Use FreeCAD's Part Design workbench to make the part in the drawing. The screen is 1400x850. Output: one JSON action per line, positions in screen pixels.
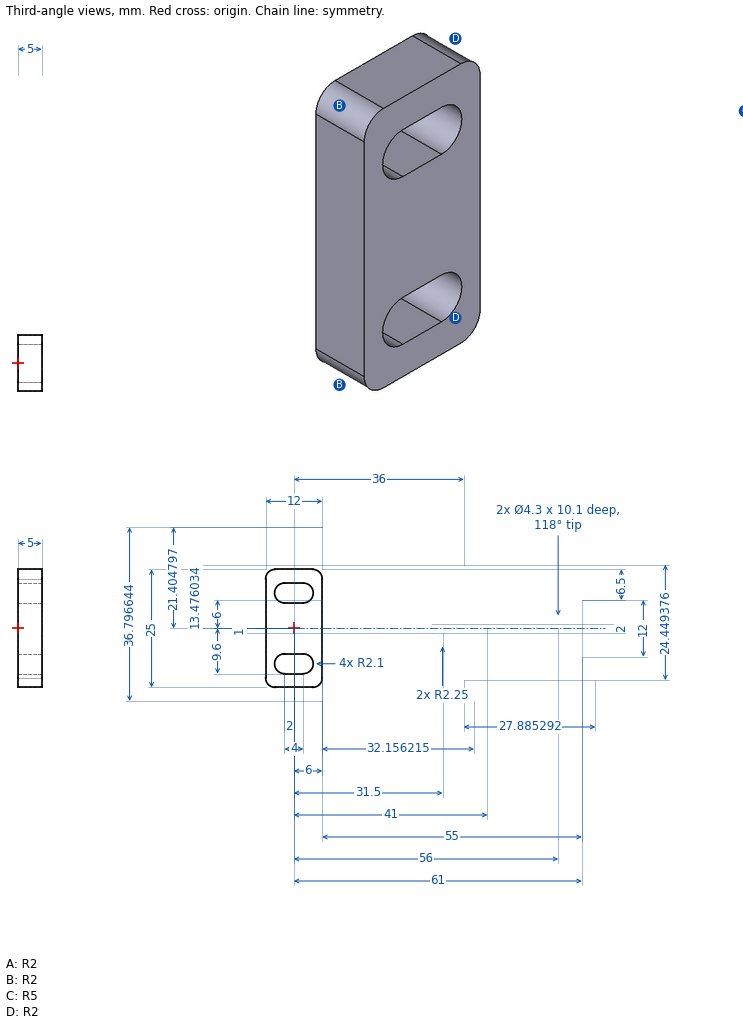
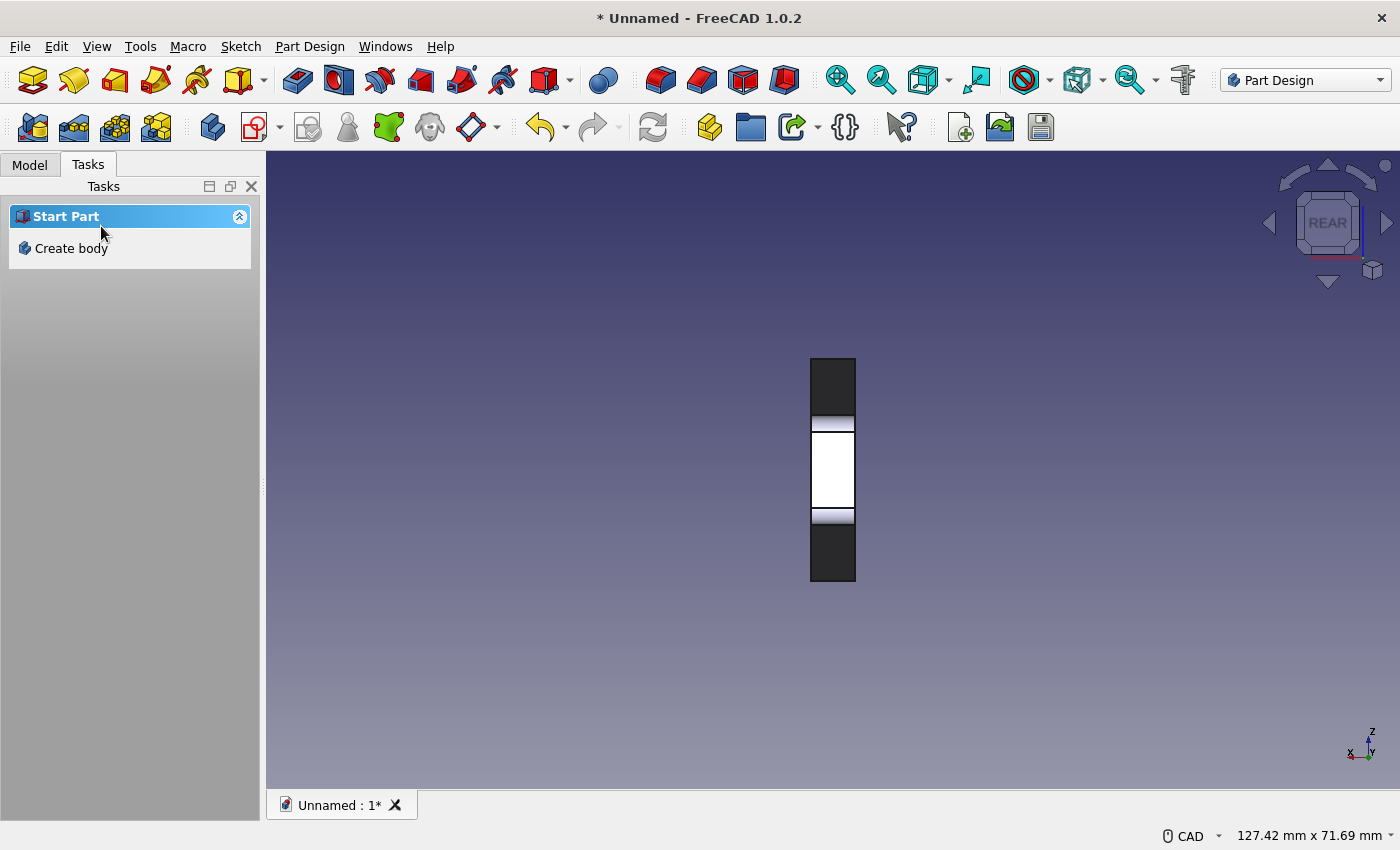
{"action": "left_click", "coordinate": [841, 80]}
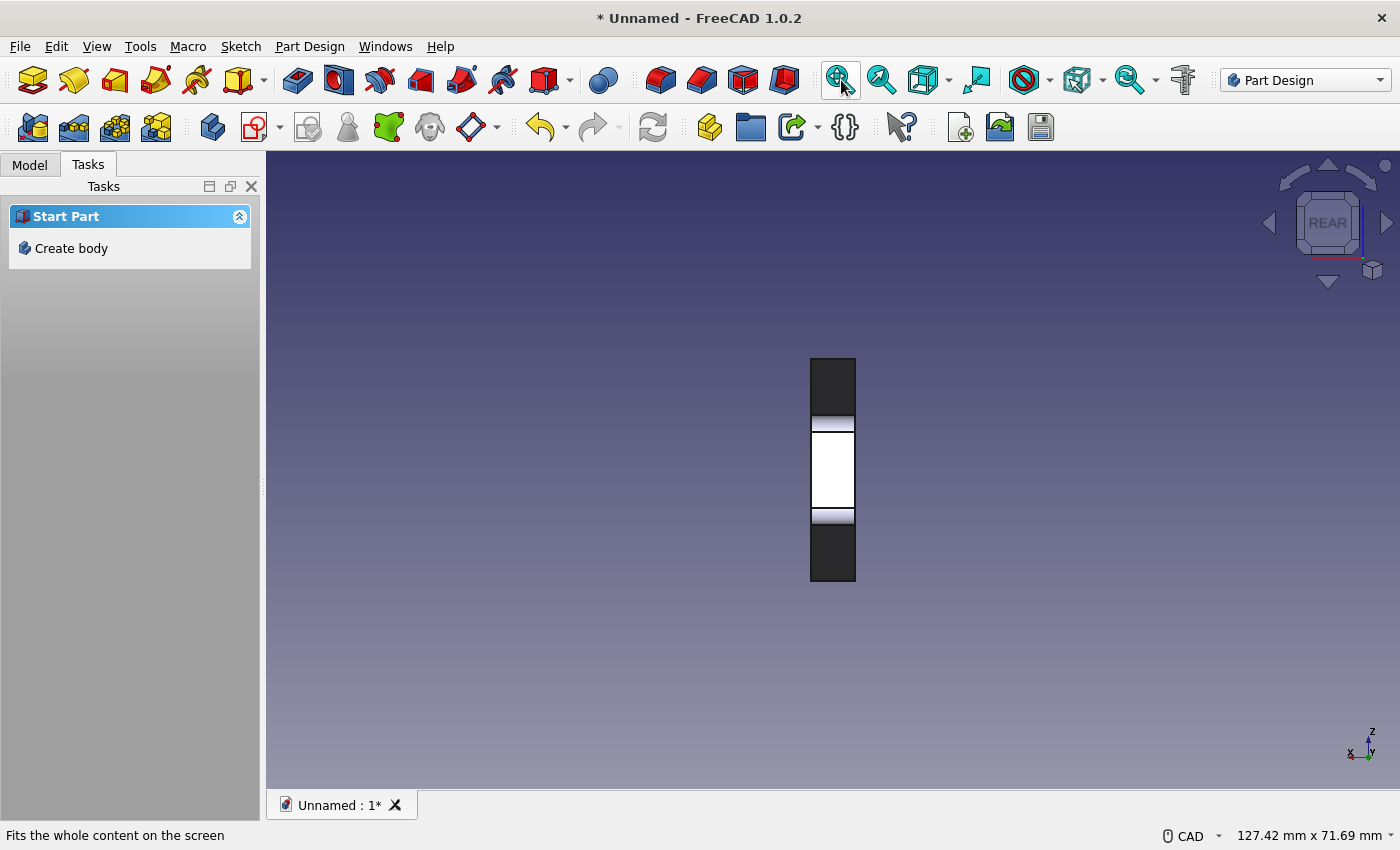
{"action": "key", "text": "6"}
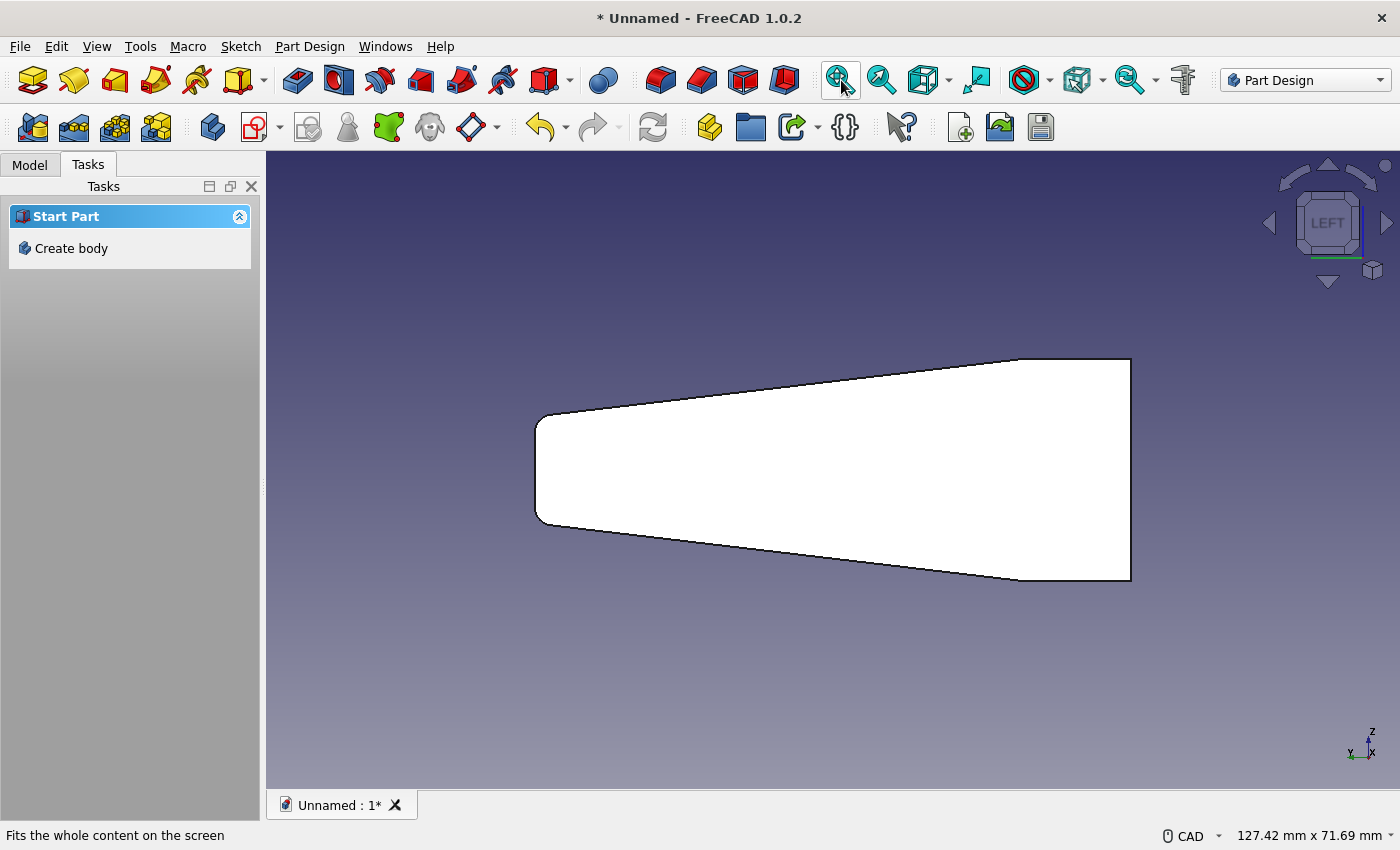
{"action": "left_click", "coordinate": [1003, 469]}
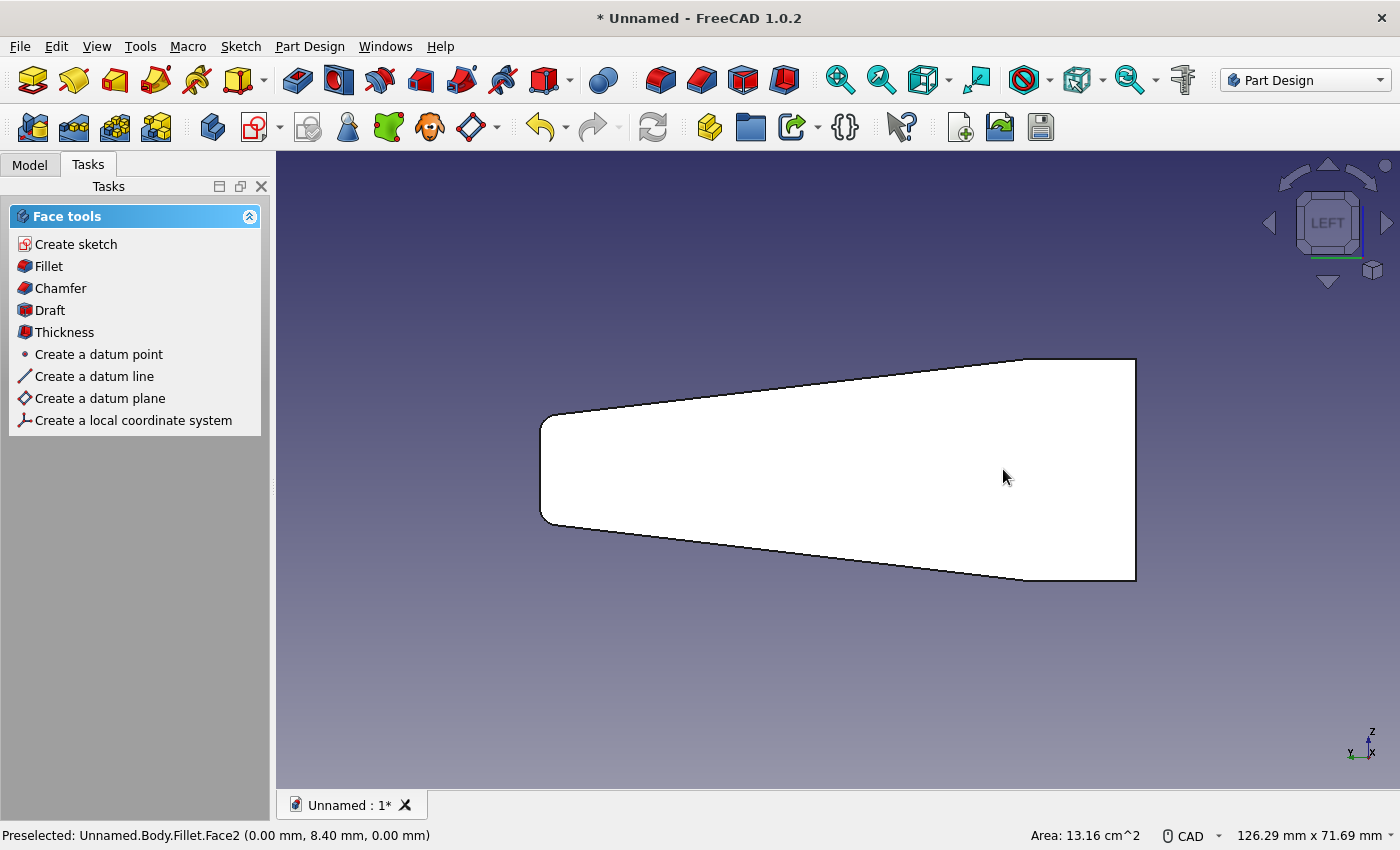
{"action": "left_click", "coordinate": [254, 128]}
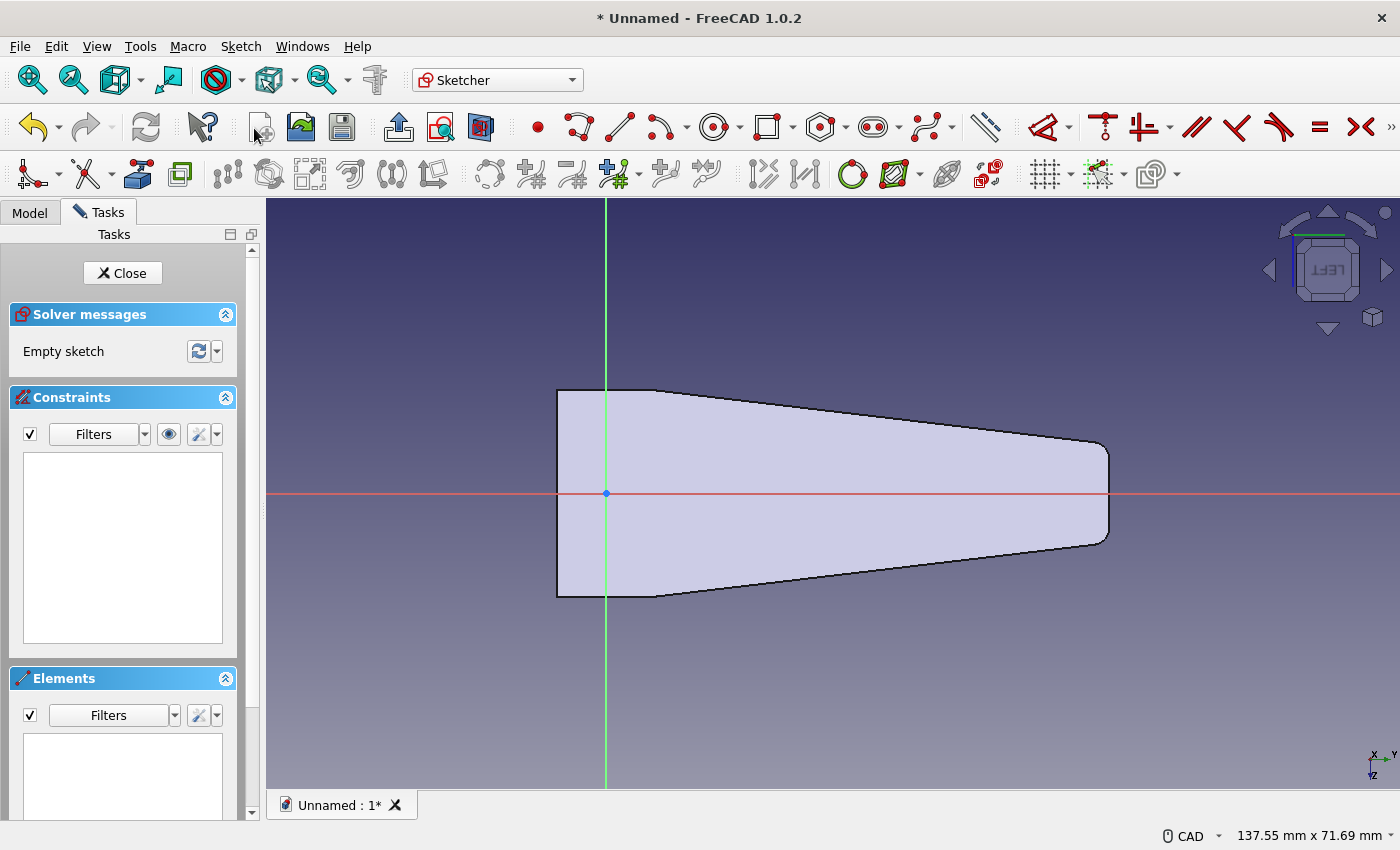
{"action": "scroll", "coordinate": [477, 494], "scroll_direction": "up", "scroll_amount": 4}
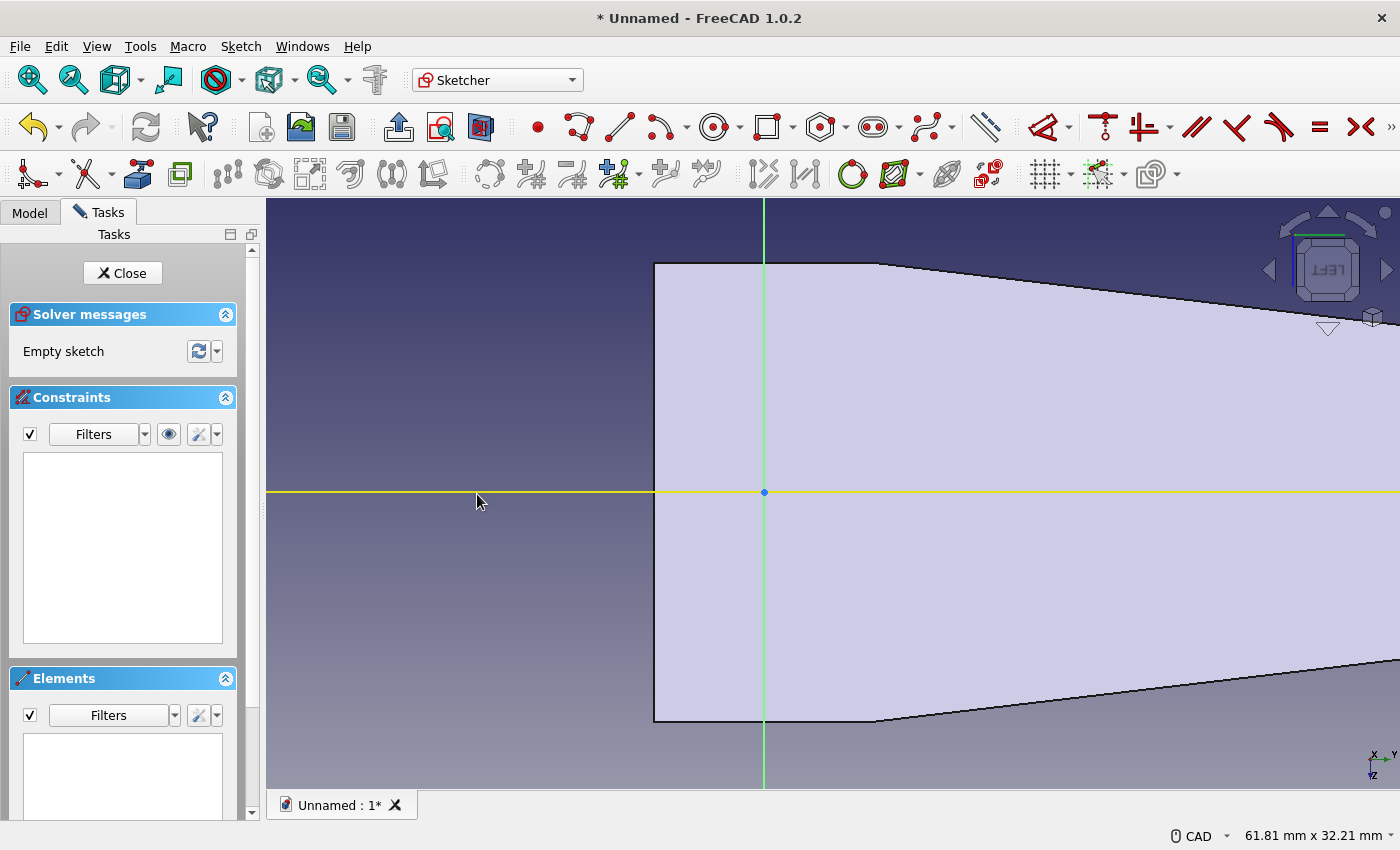
{"action": "left_click", "coordinate": [872, 128]}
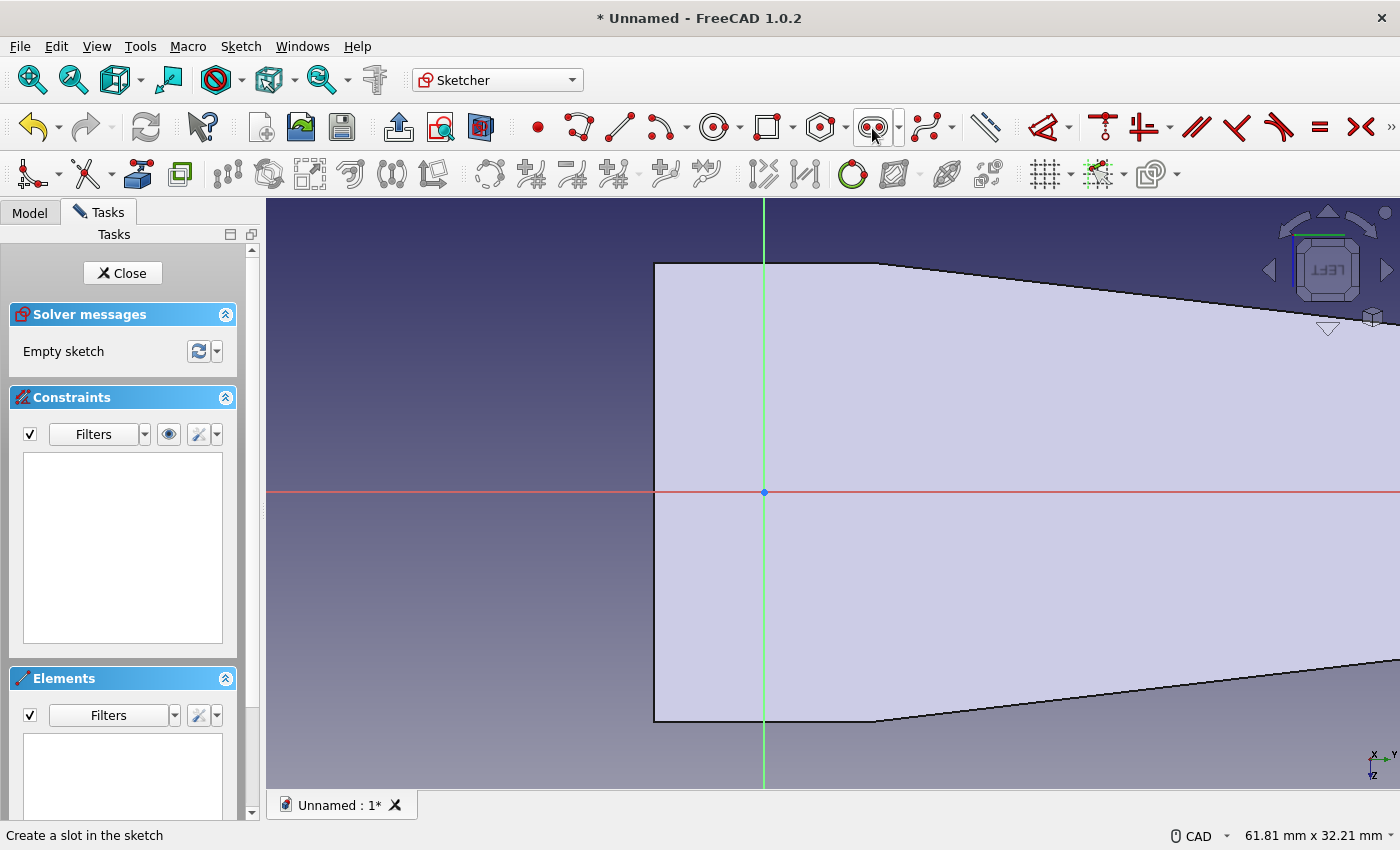
{"action": "left_click", "coordinate": [728, 355]}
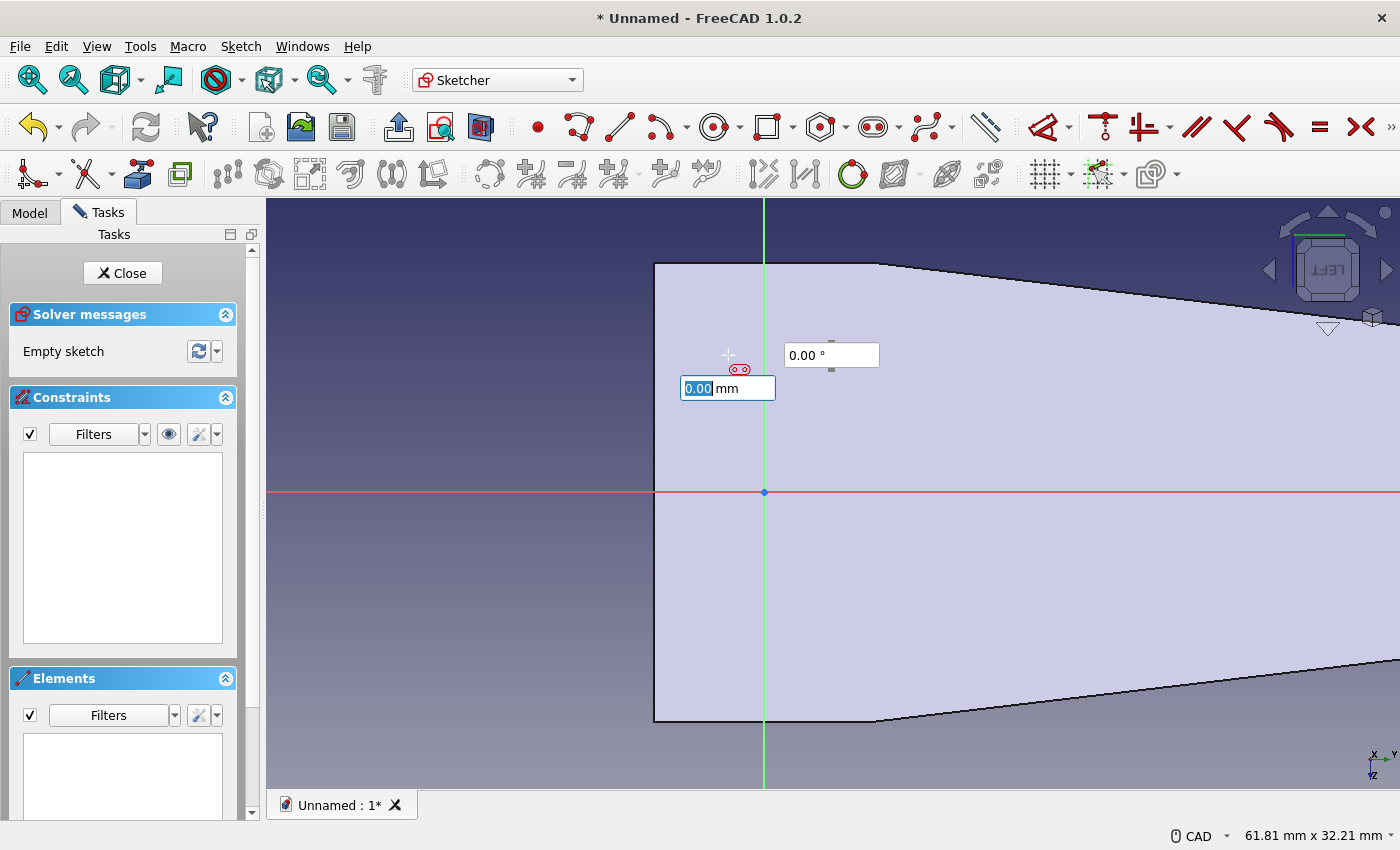
{"action": "left_click", "coordinate": [801, 355]}